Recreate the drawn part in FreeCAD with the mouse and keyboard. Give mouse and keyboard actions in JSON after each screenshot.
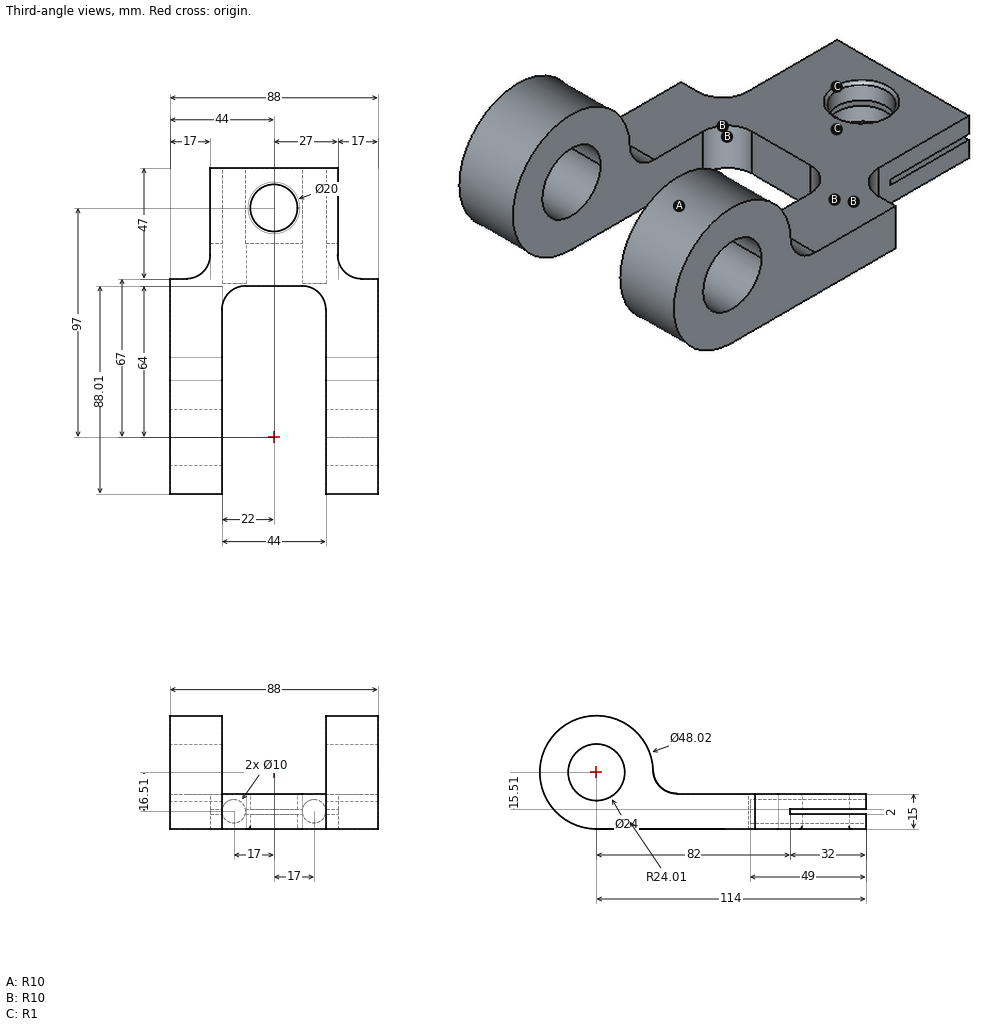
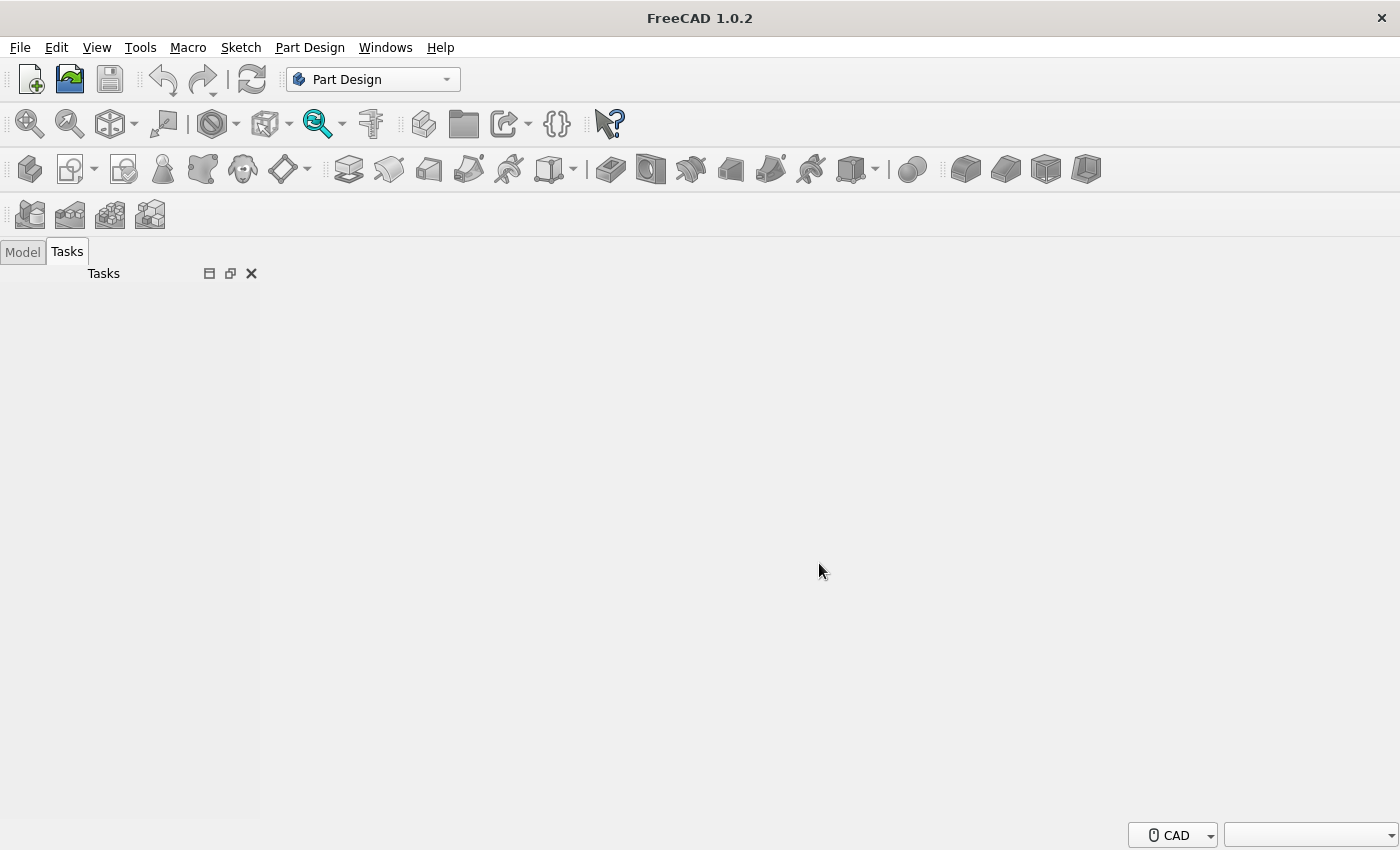
{"action": "left_click", "coordinate": [30, 80]}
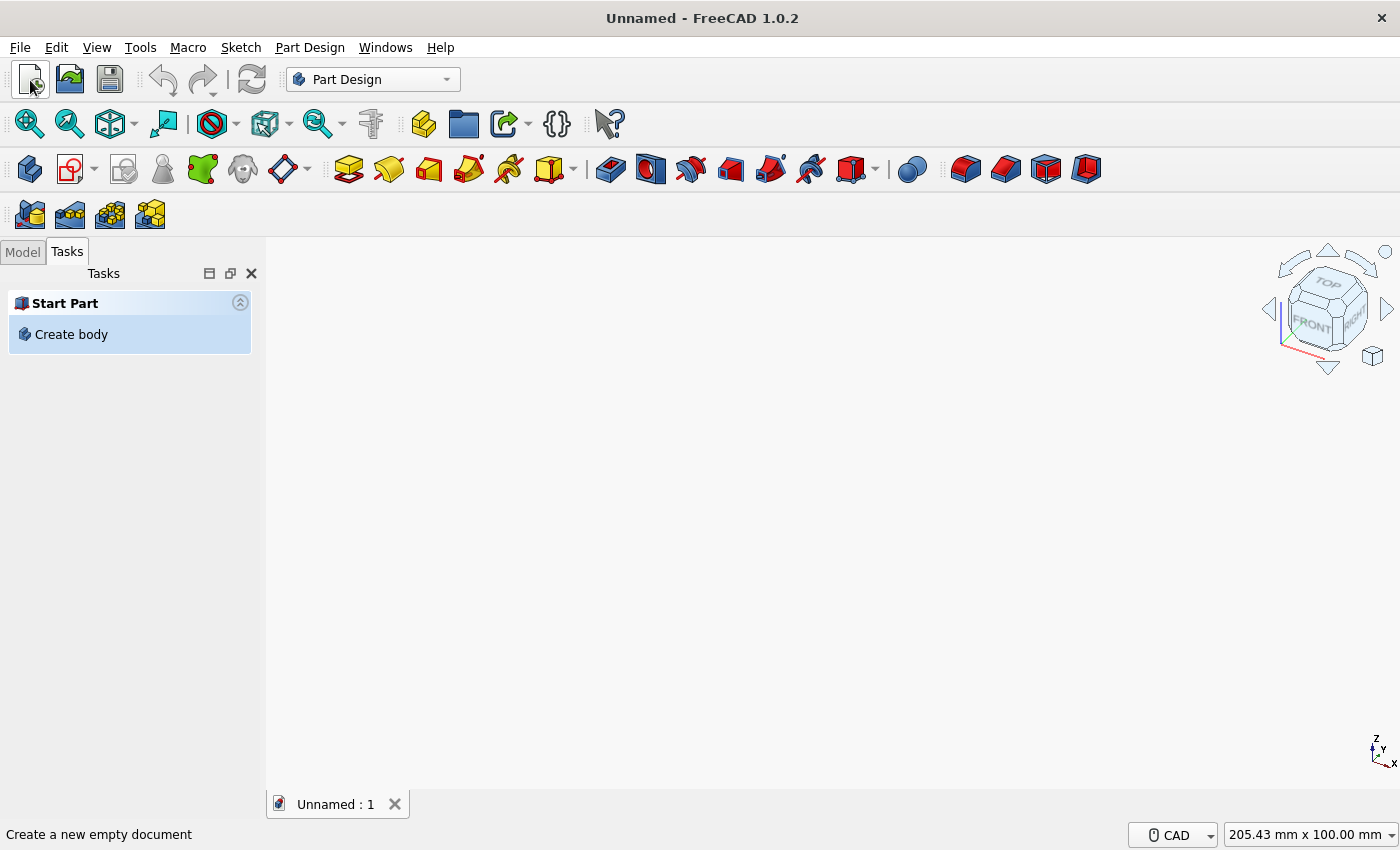
{"action": "left_click", "coordinate": [70, 170]}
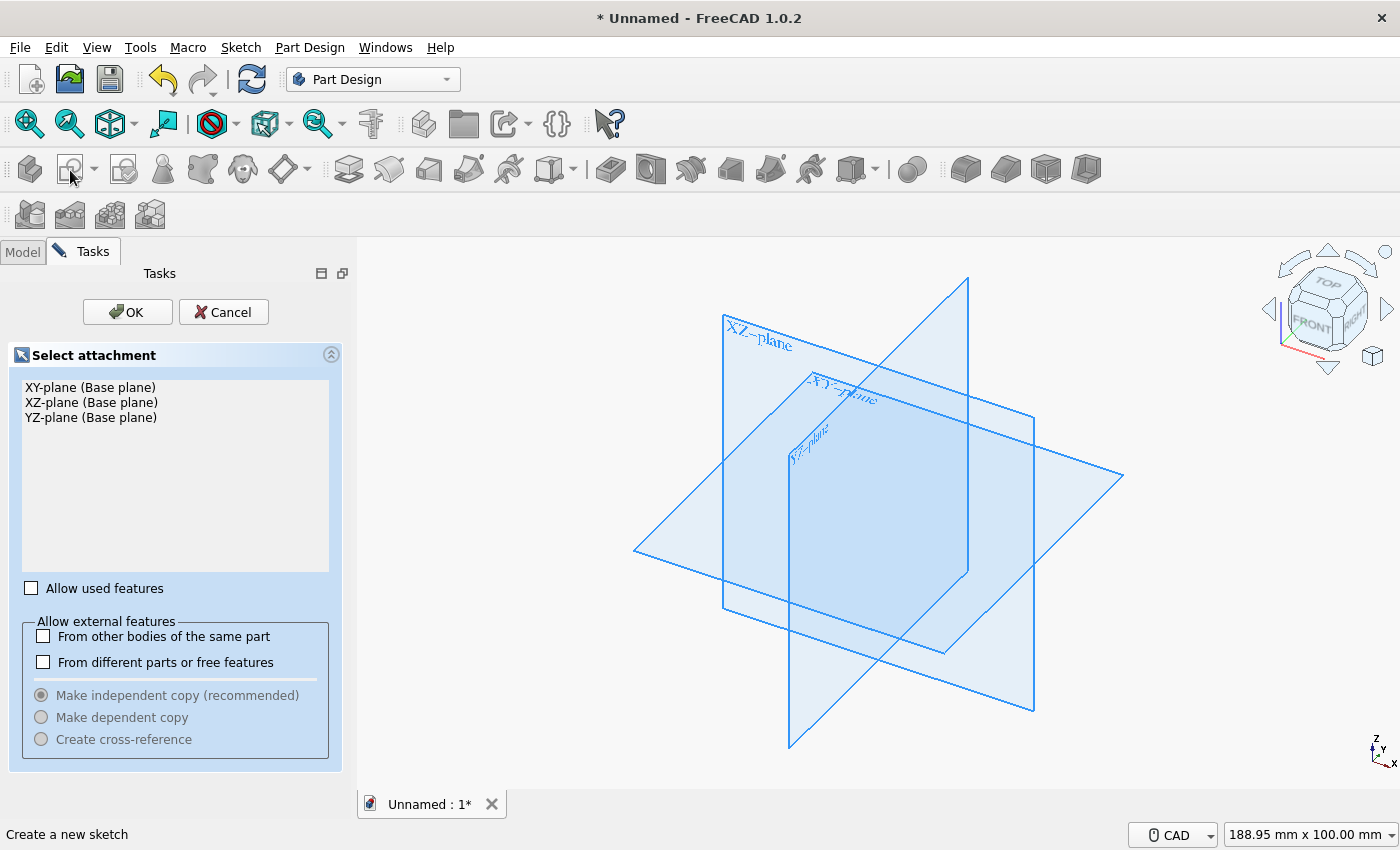
{"action": "left_click", "coordinate": [82, 418]}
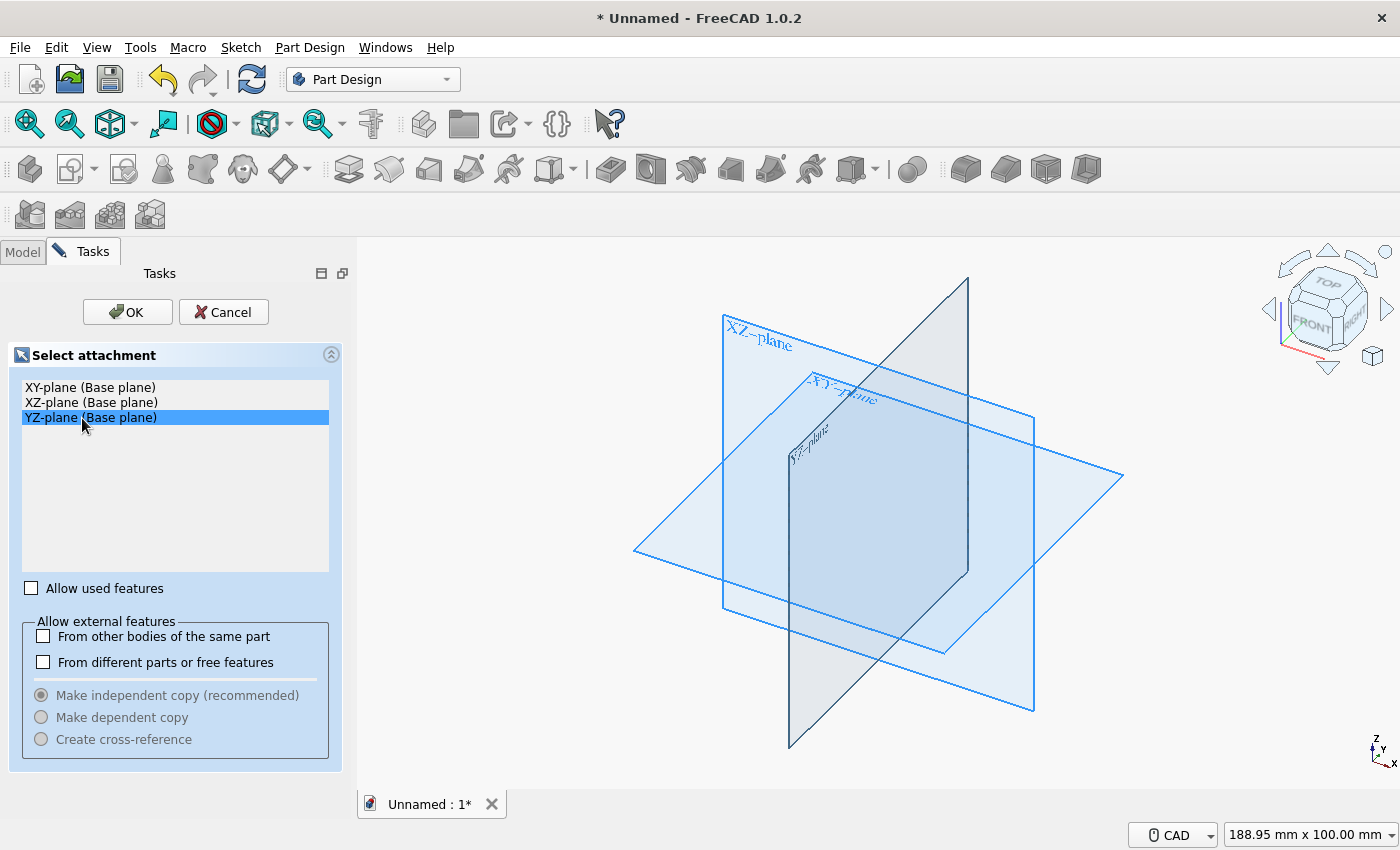
{"action": "left_click", "coordinate": [128, 312]}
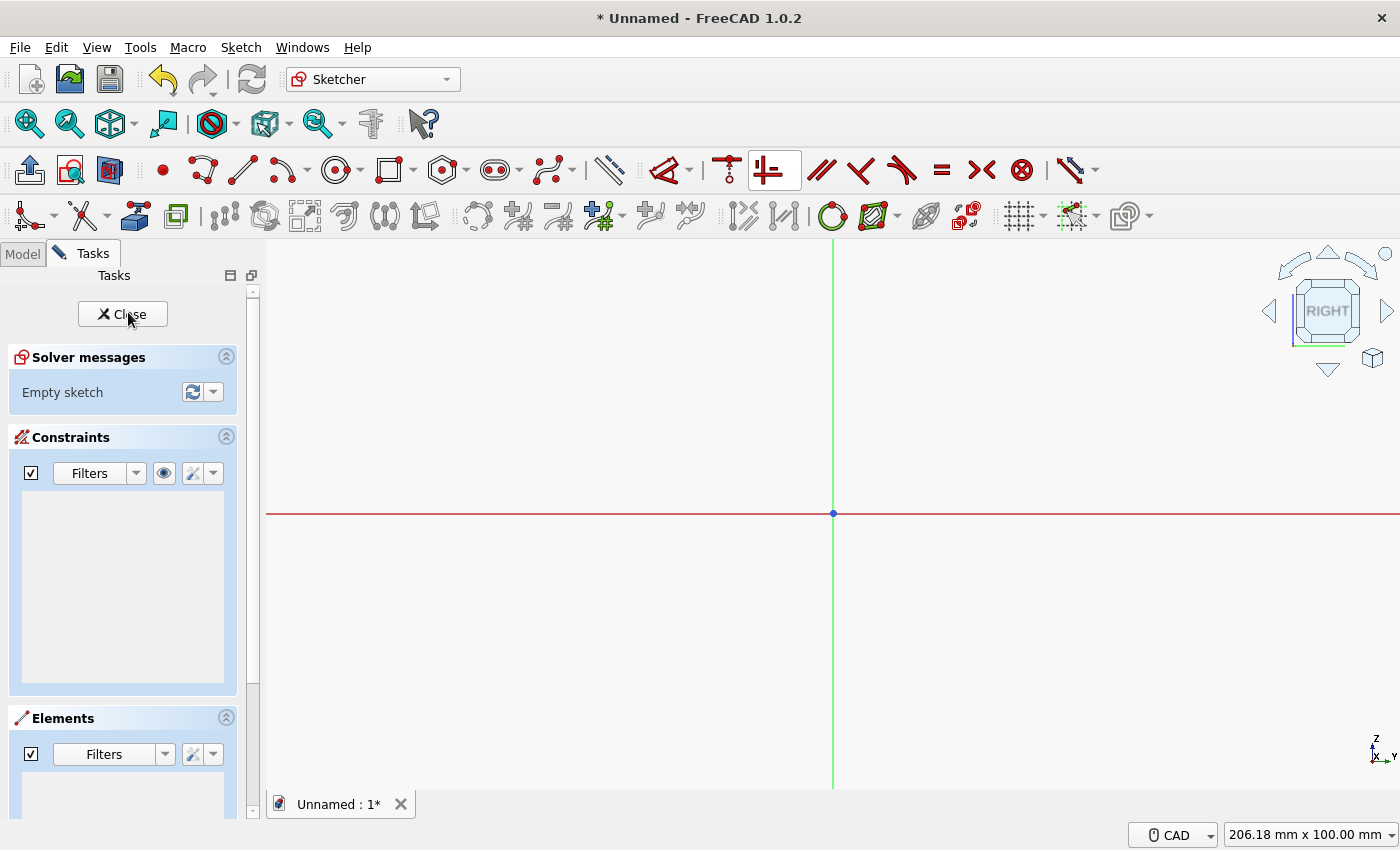
{"action": "left_click", "coordinate": [336, 170]}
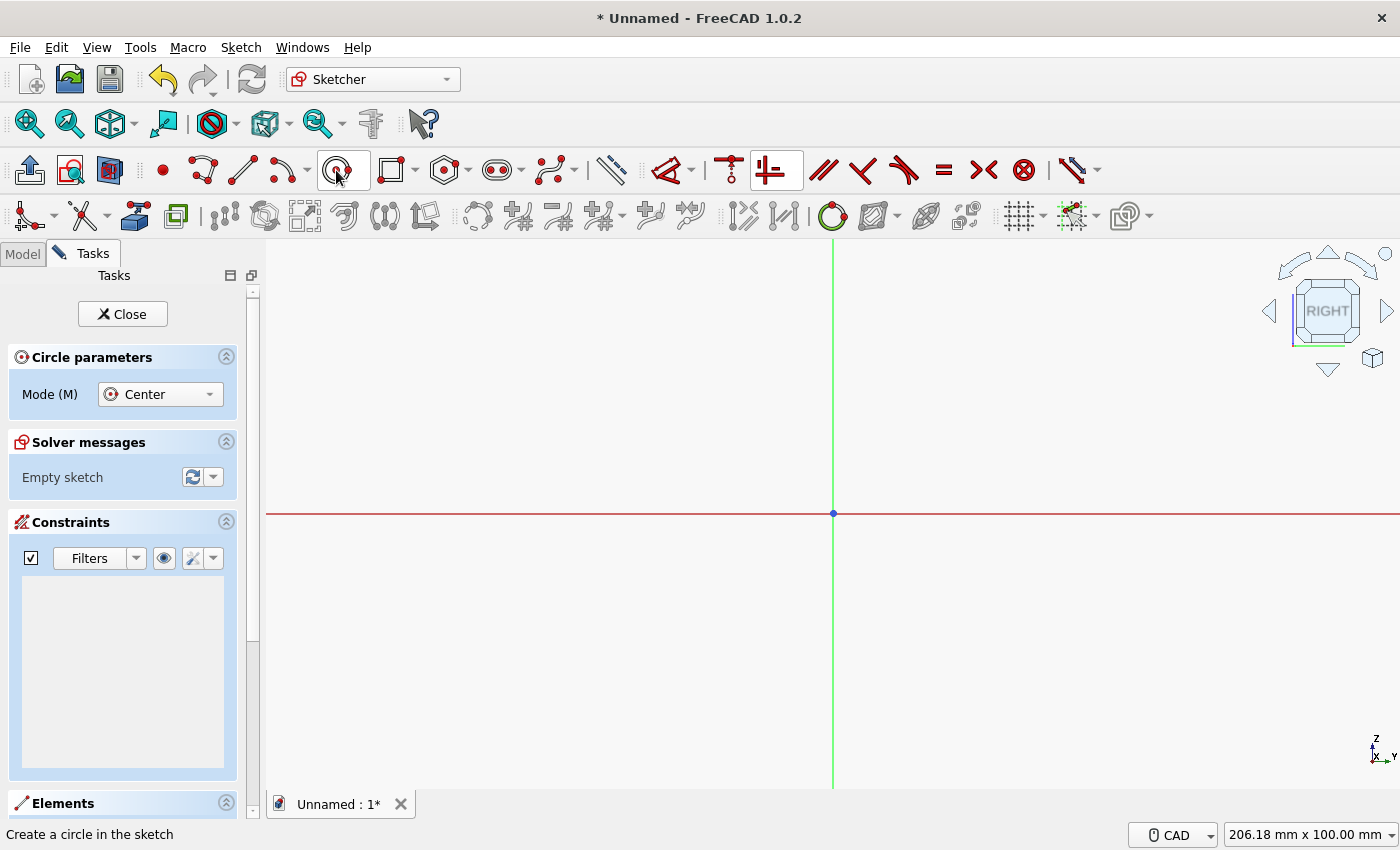
{"action": "left_click", "coordinate": [833, 514]}
{"action": "left_click", "coordinate": [926, 421]}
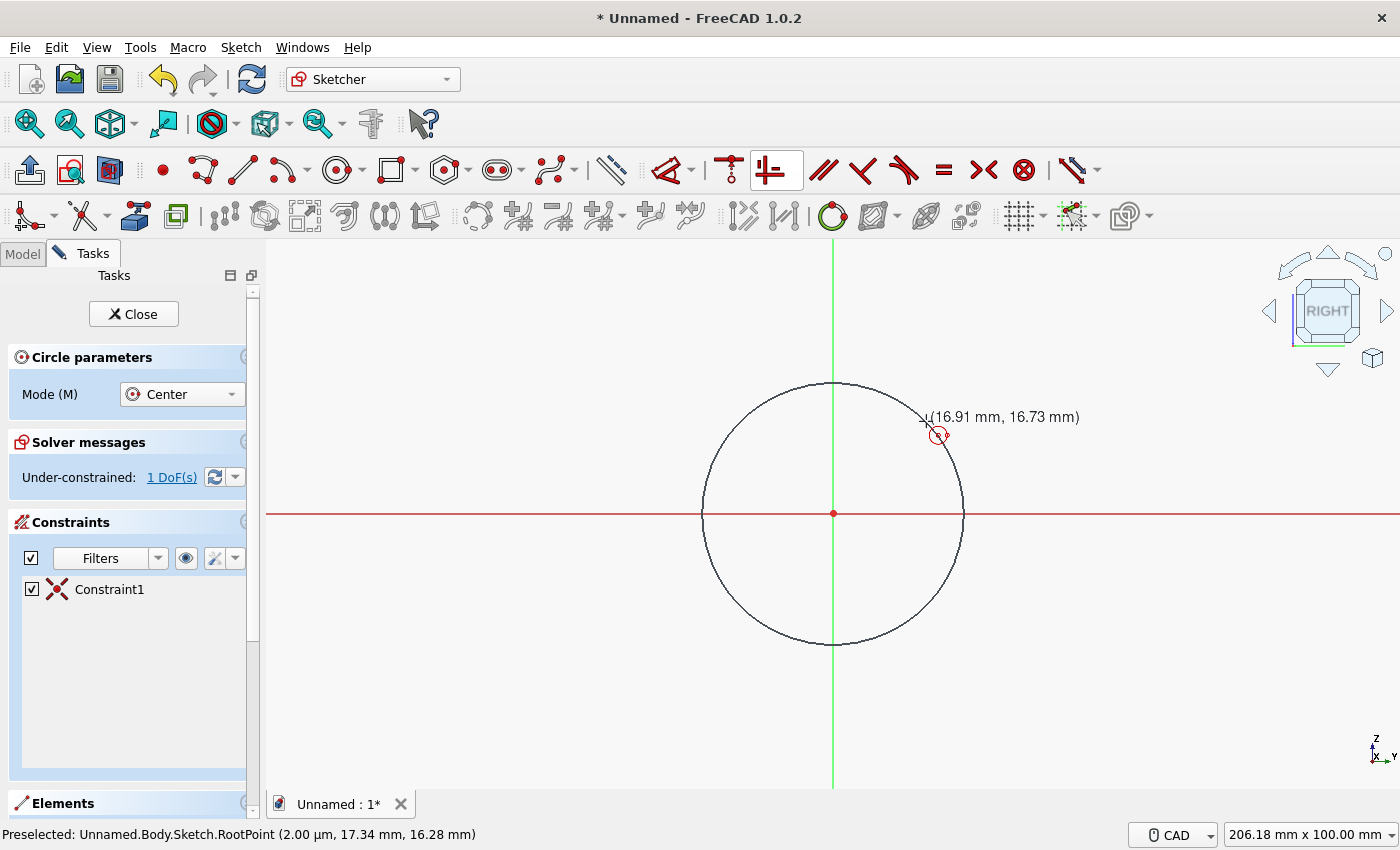
{"action": "left_click", "coordinate": [833, 514]}
{"action": "left_click", "coordinate": [880, 467]}
{"action": "key", "text": "Escape"}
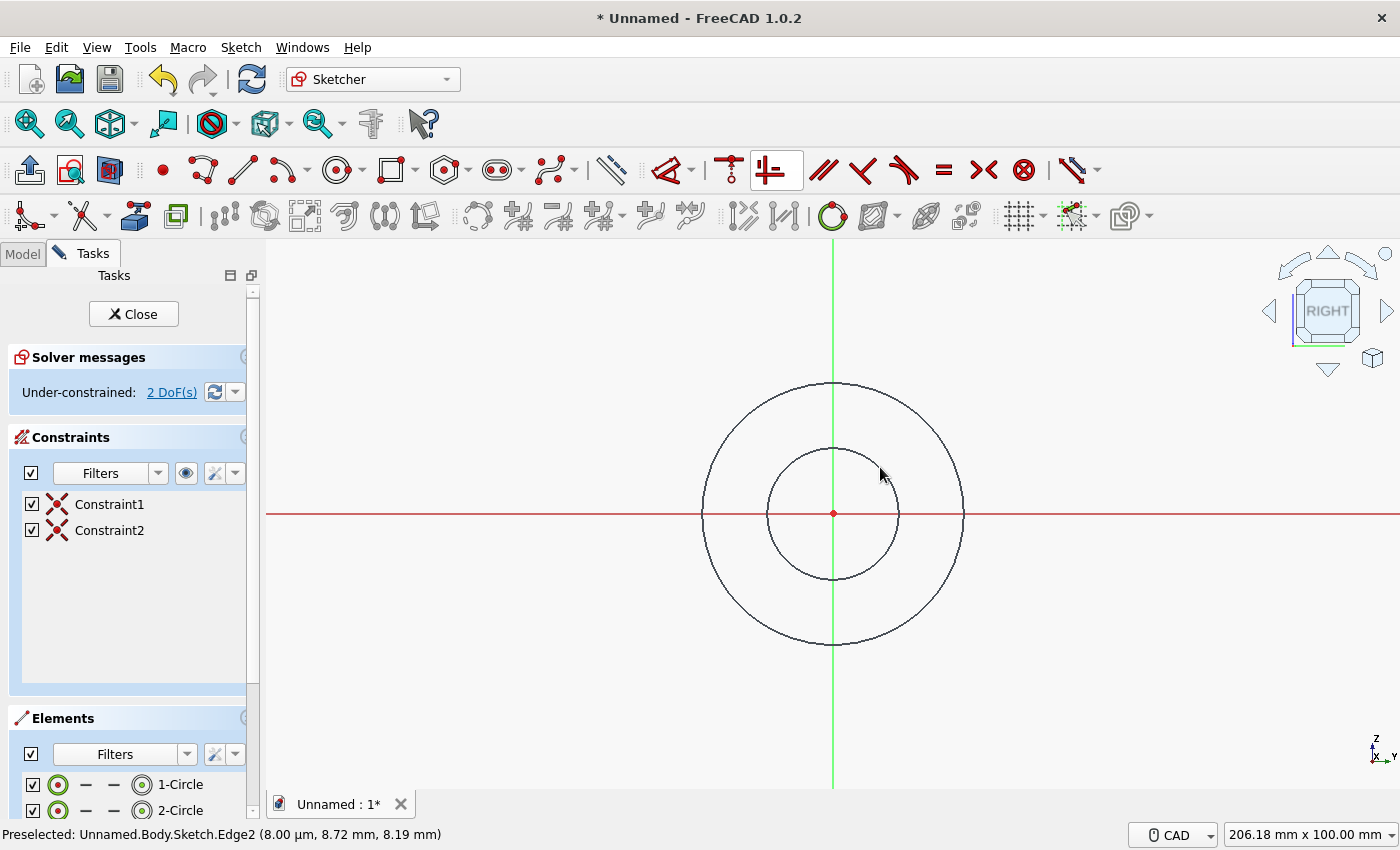
{"action": "left_click", "coordinate": [666, 170]}